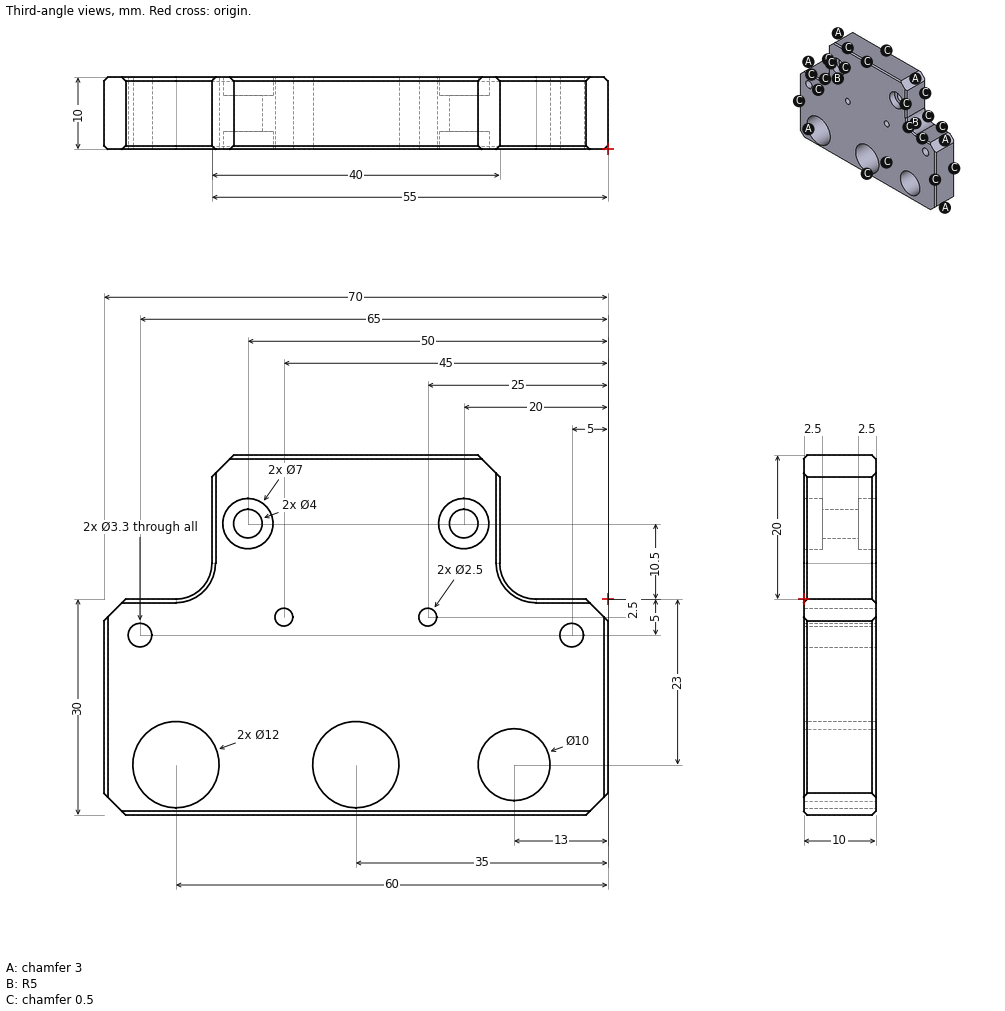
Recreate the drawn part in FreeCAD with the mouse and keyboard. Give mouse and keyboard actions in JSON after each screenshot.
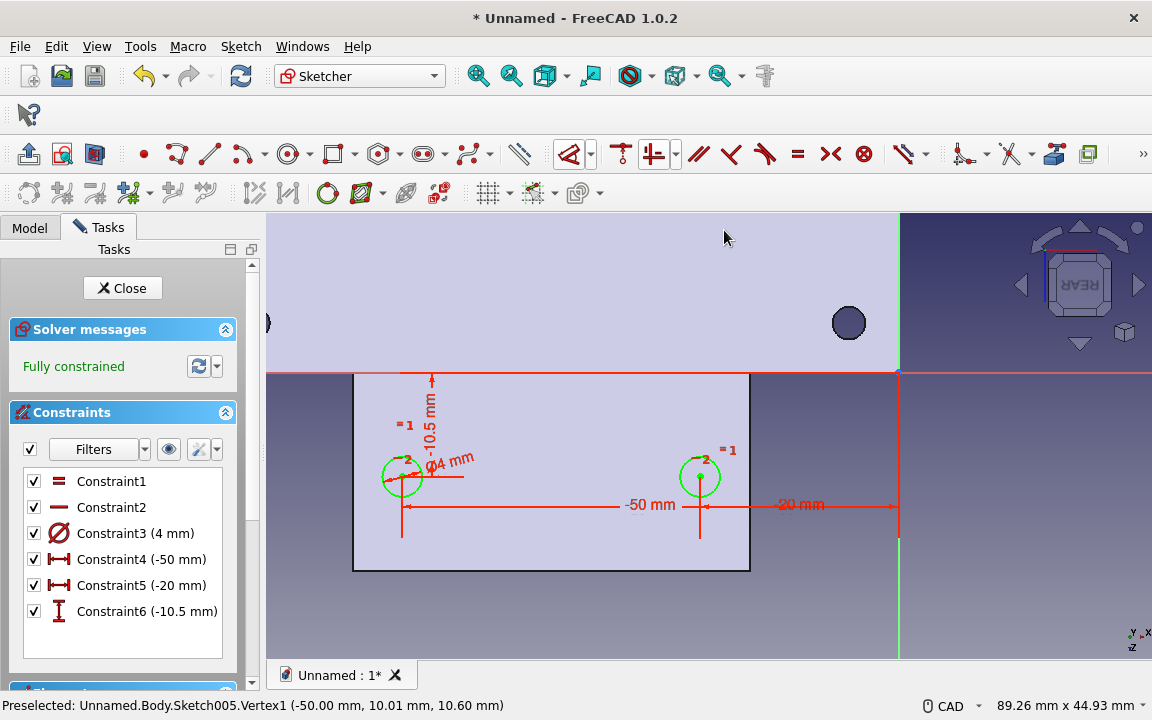
{"action": "left_click", "coordinate": [123, 288]}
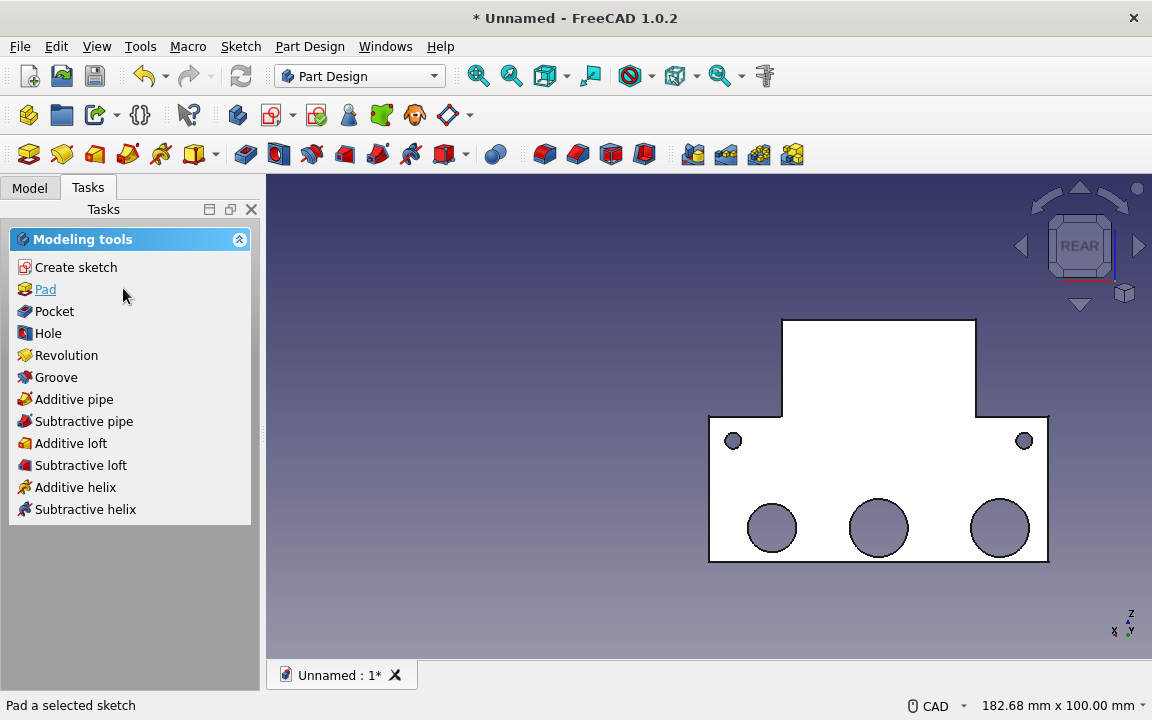
{"action": "left_click", "coordinate": [246, 154]}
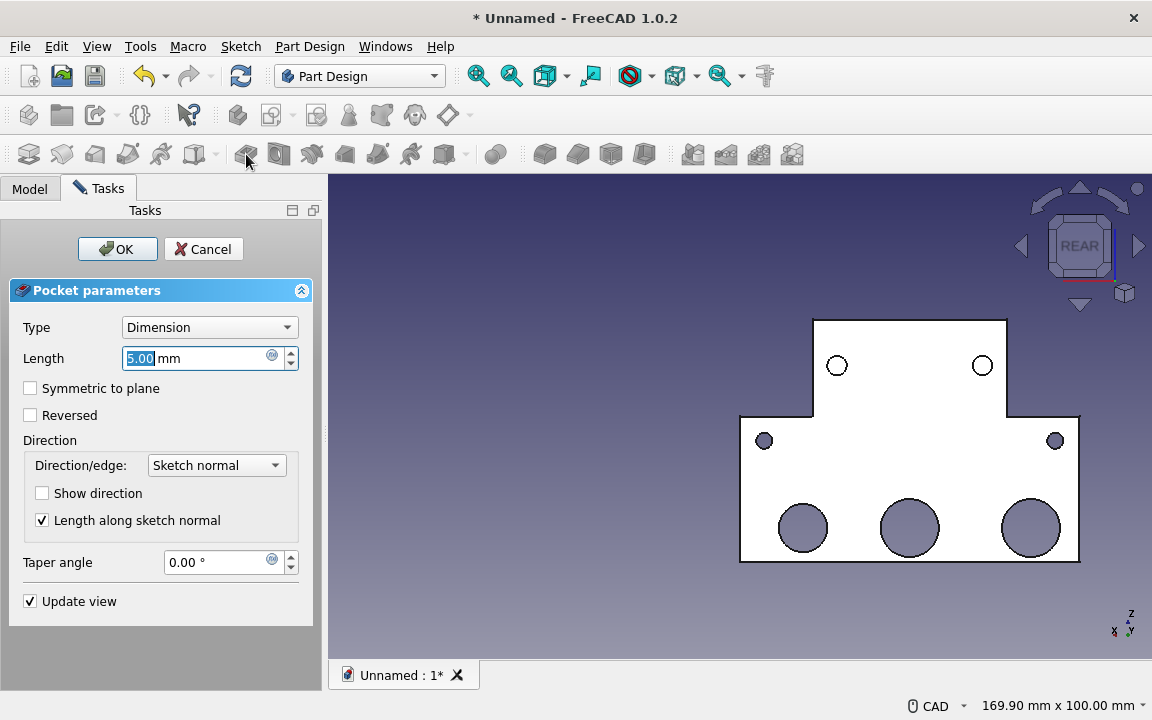
{"action": "left_click", "coordinate": [210, 328]}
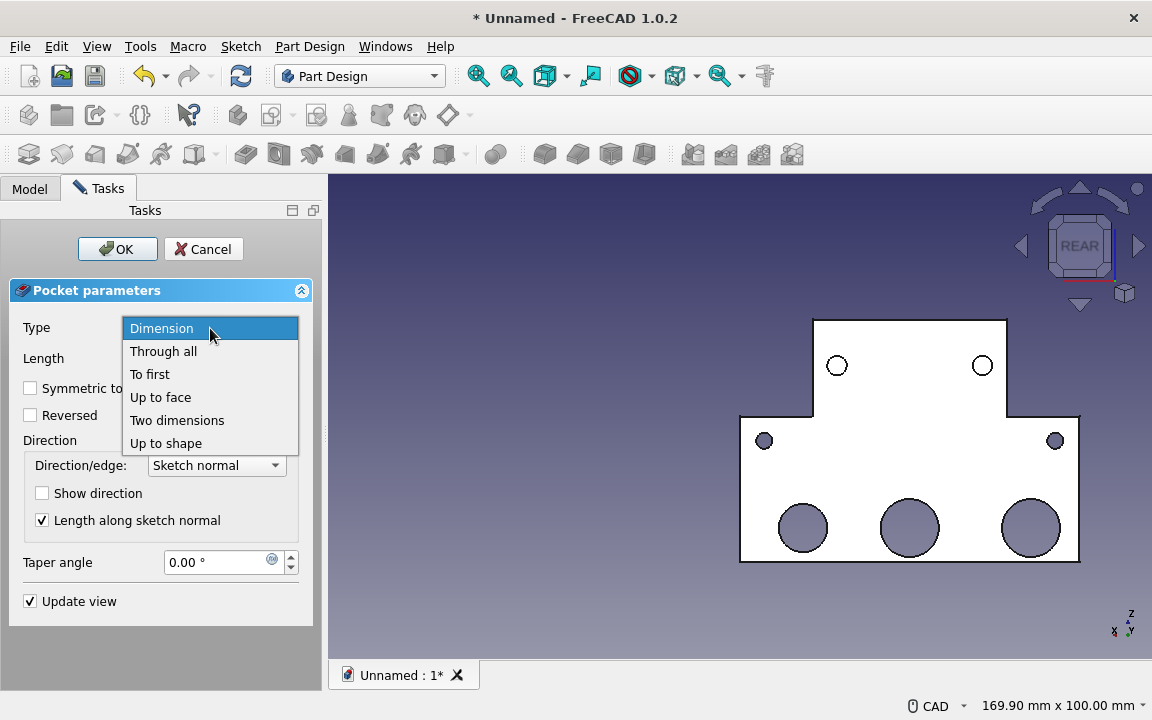
{"action": "left_click", "coordinate": [208, 352]}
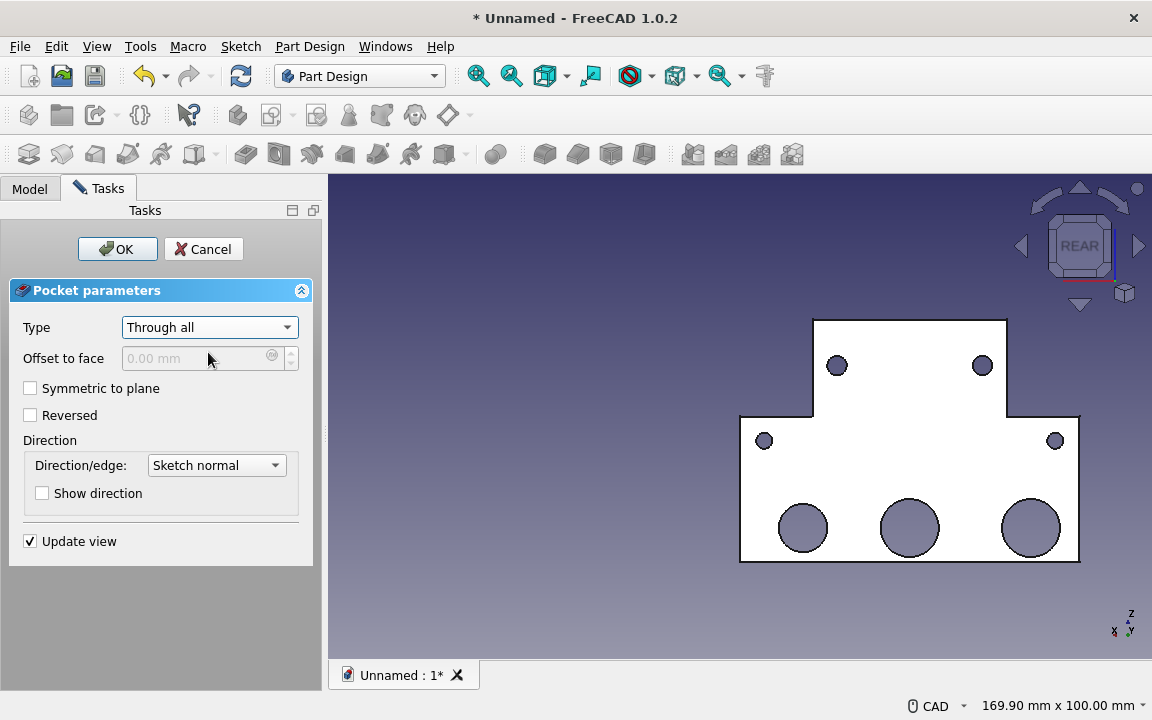
{"action": "left_click", "coordinate": [118, 249]}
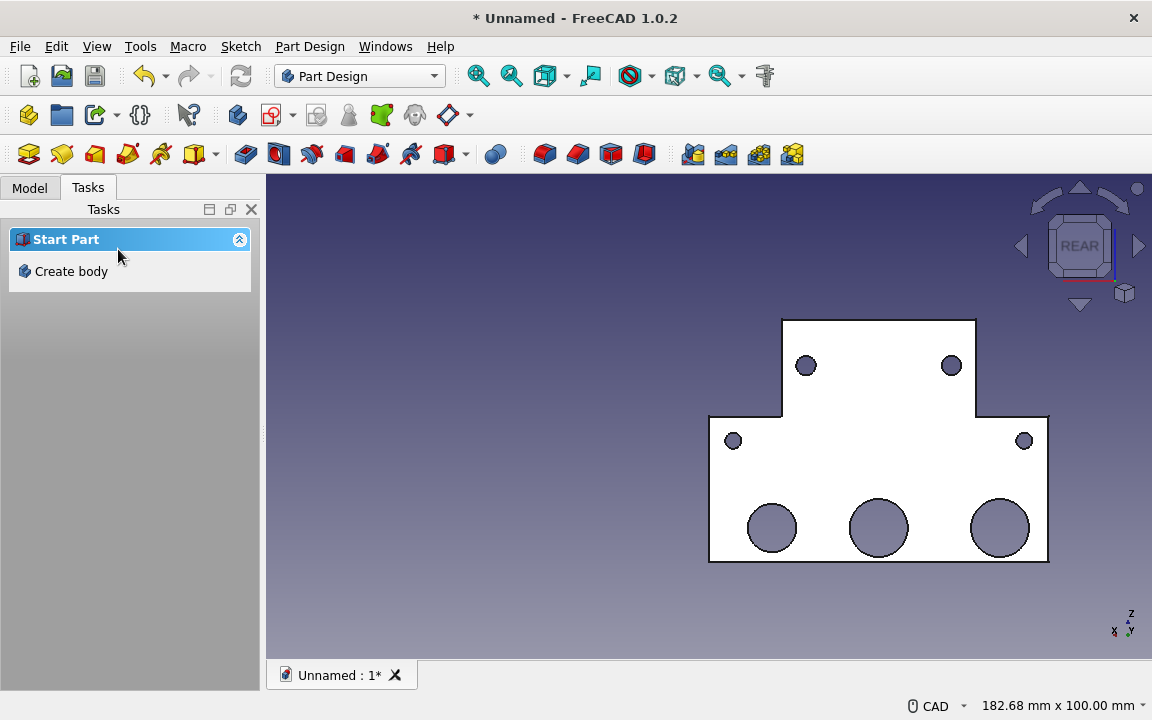
{"action": "left_click", "coordinate": [270, 116]}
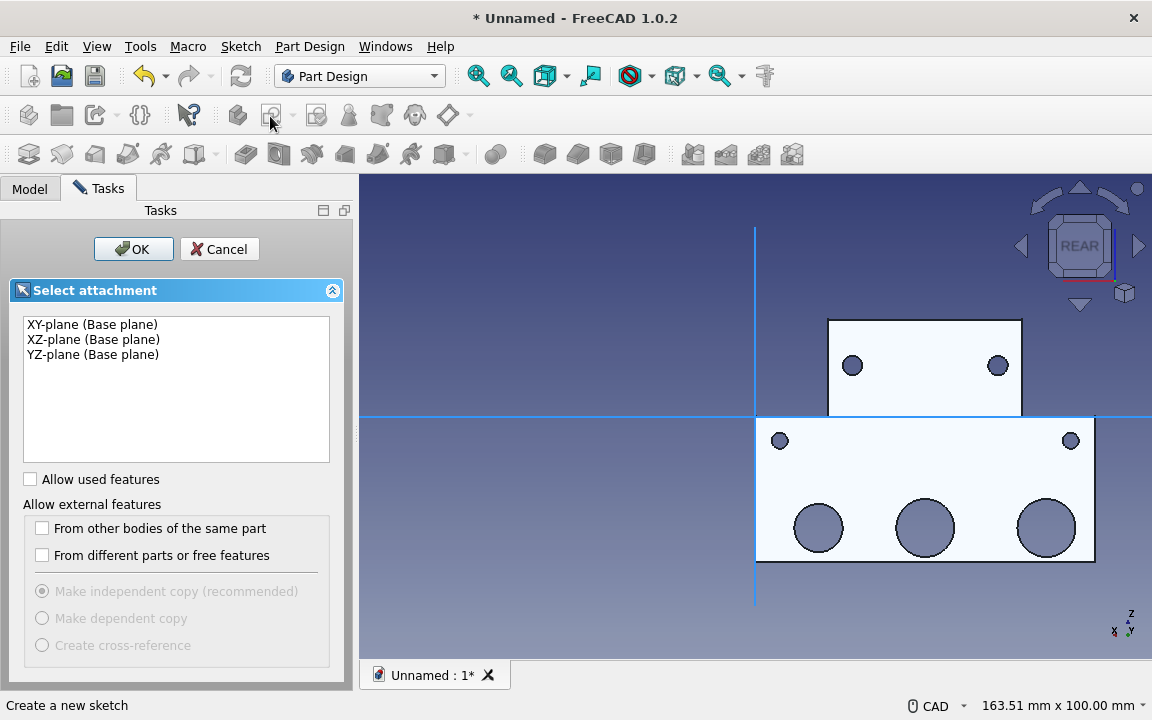
{"action": "left_click", "coordinate": [84, 340]}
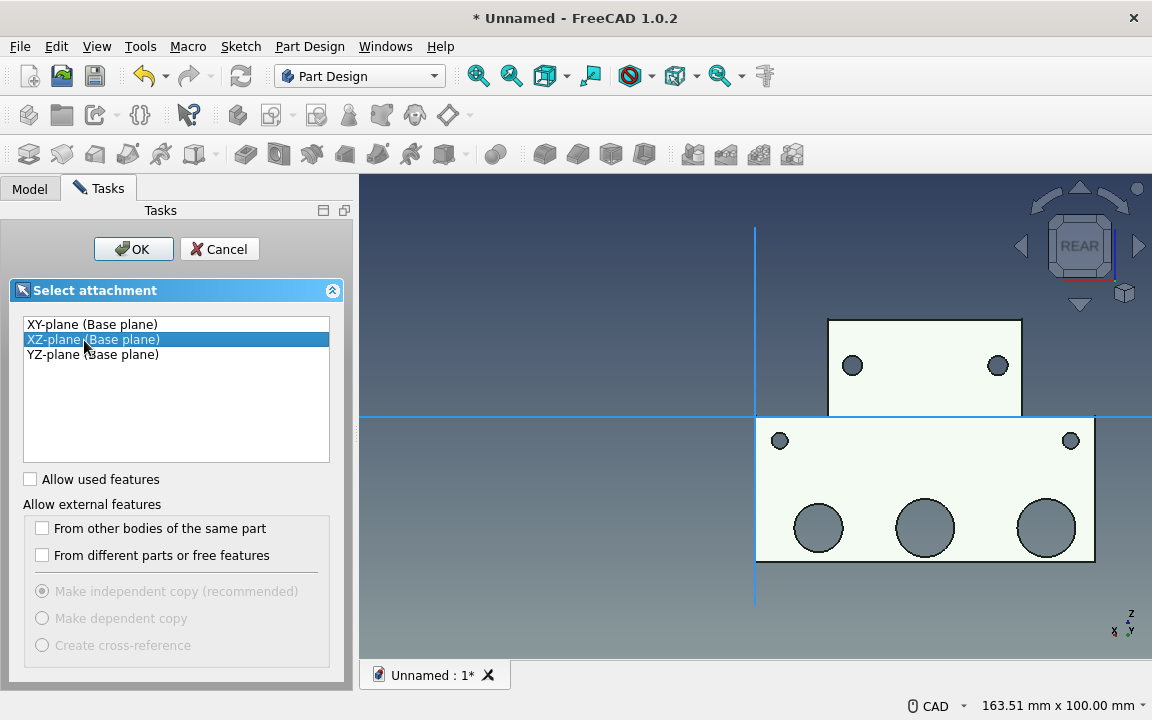
{"action": "left_click", "coordinate": [134, 249]}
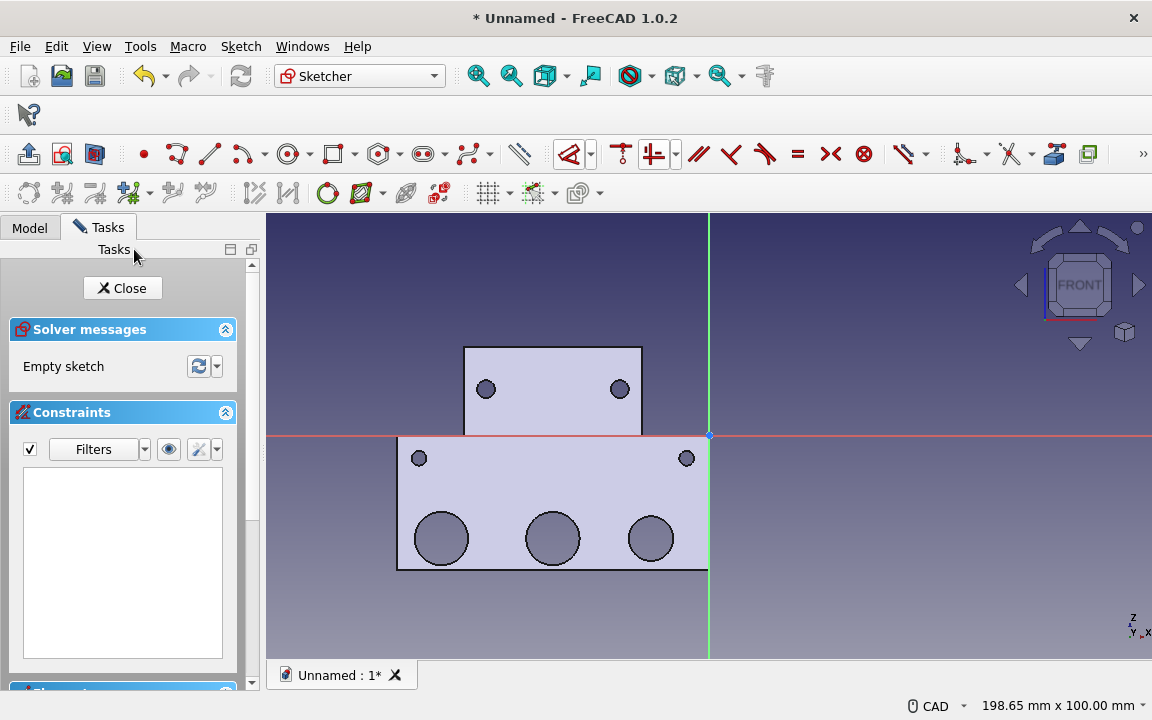
{"action": "scroll", "coordinate": [578, 451], "scroll_direction": "up", "scroll_amount": 4}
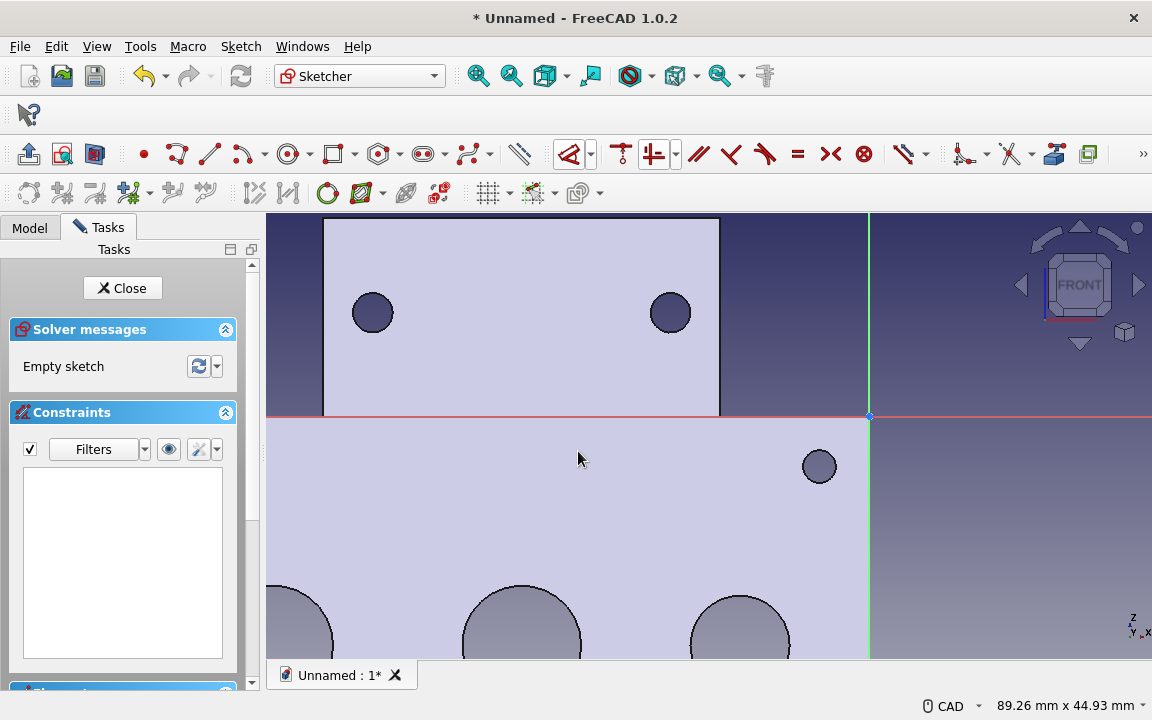
{"action": "left_click", "coordinate": [288, 154]}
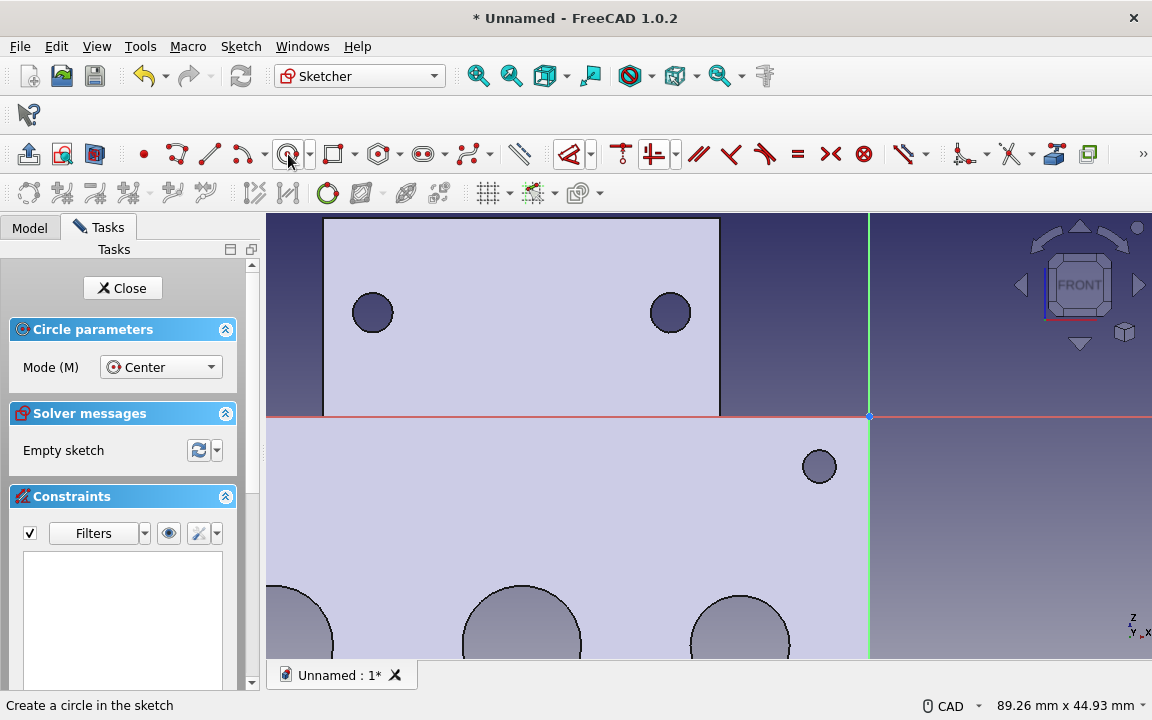
{"action": "scroll", "coordinate": [621, 442], "scroll_direction": "up", "scroll_amount": 4}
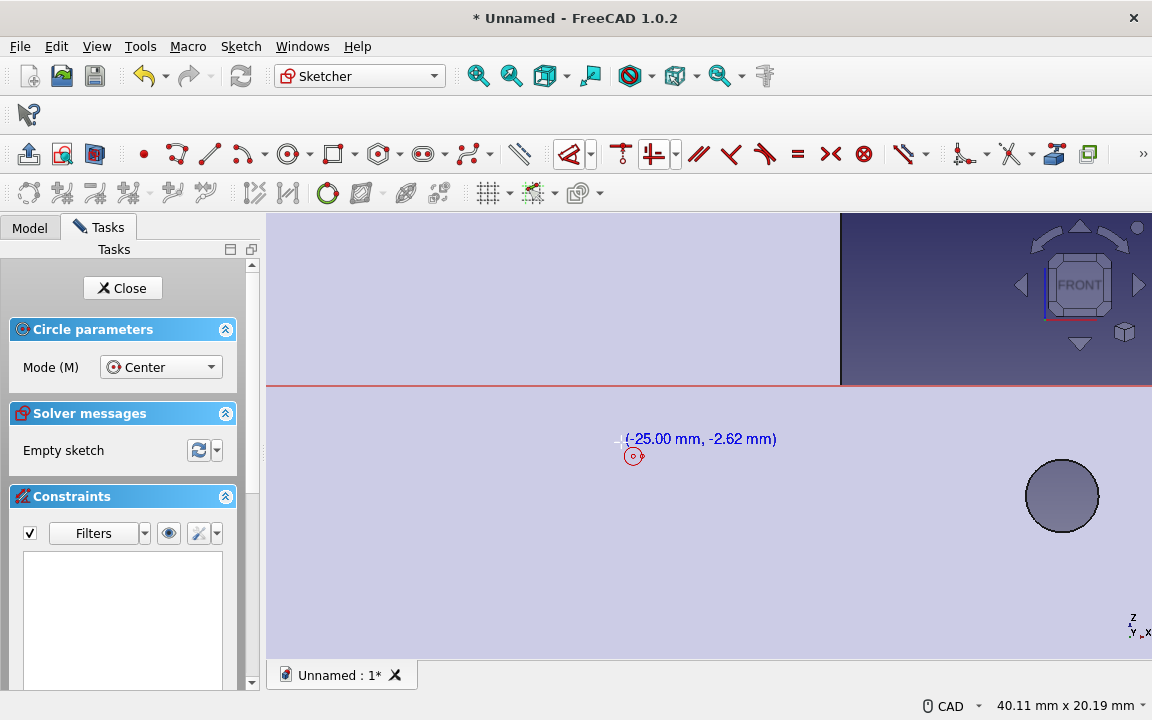
{"action": "left_click", "coordinate": [620, 441]}
{"action": "left_click", "coordinate": [640, 421]}